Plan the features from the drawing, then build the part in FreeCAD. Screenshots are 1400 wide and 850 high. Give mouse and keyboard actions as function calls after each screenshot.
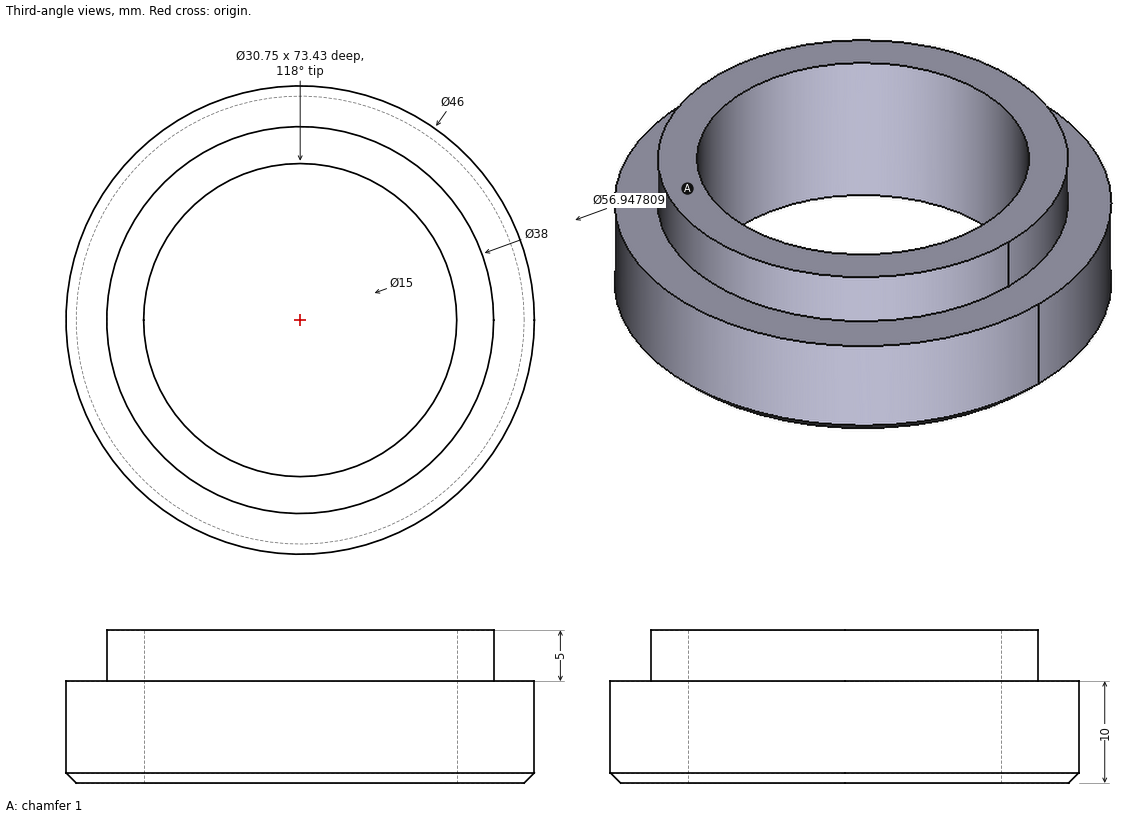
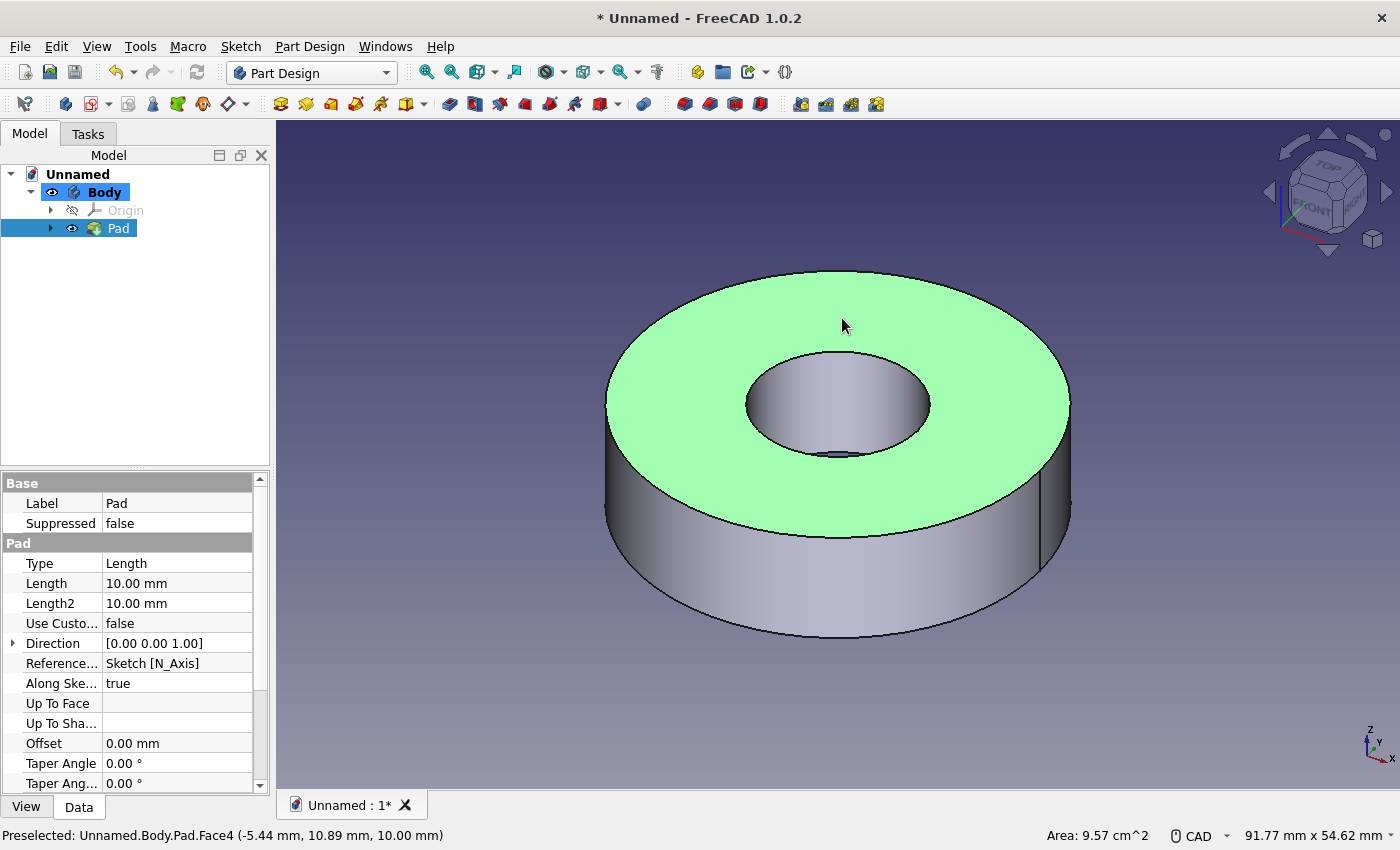
click(90, 104)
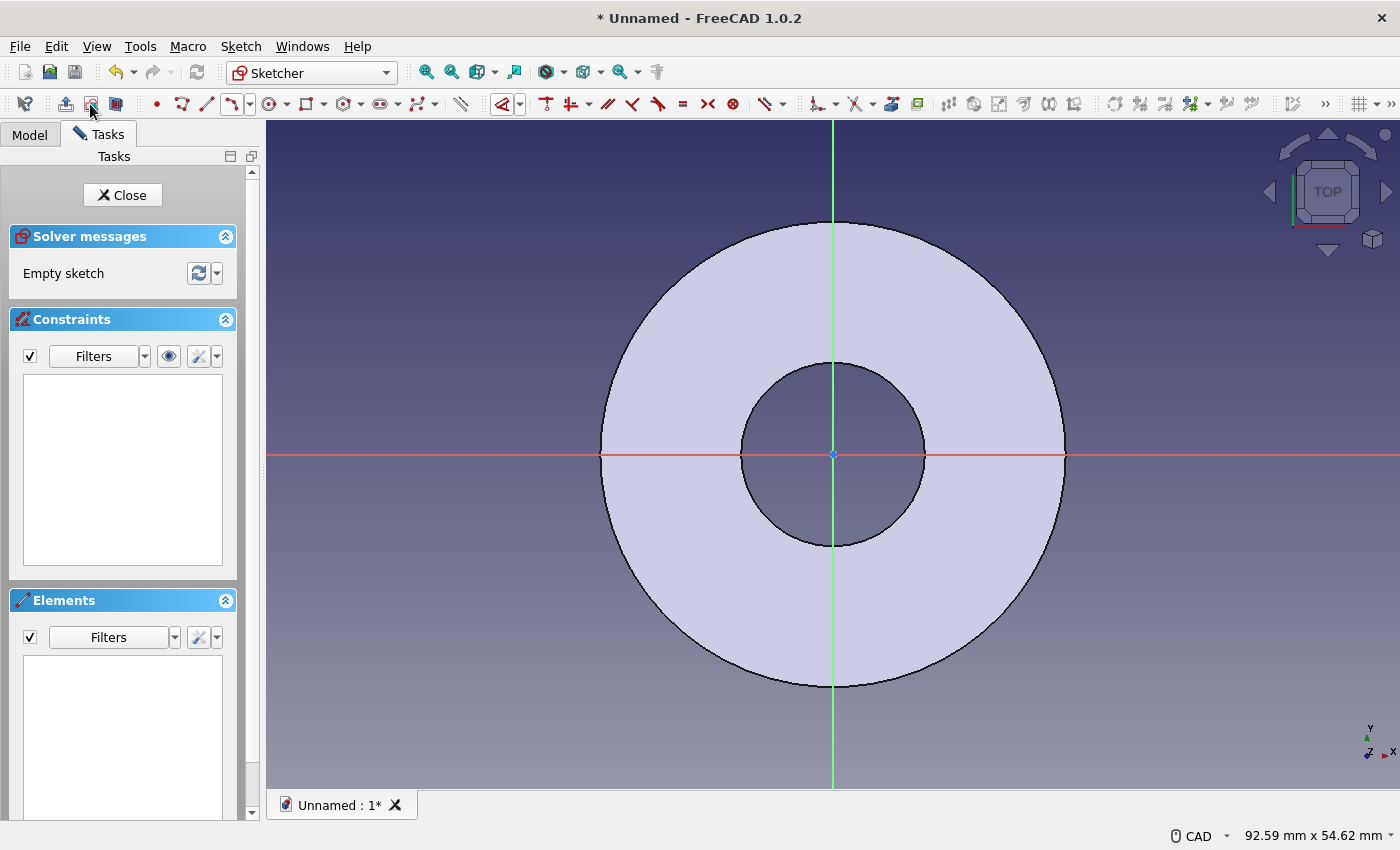
scroll(455, 455, down, 1)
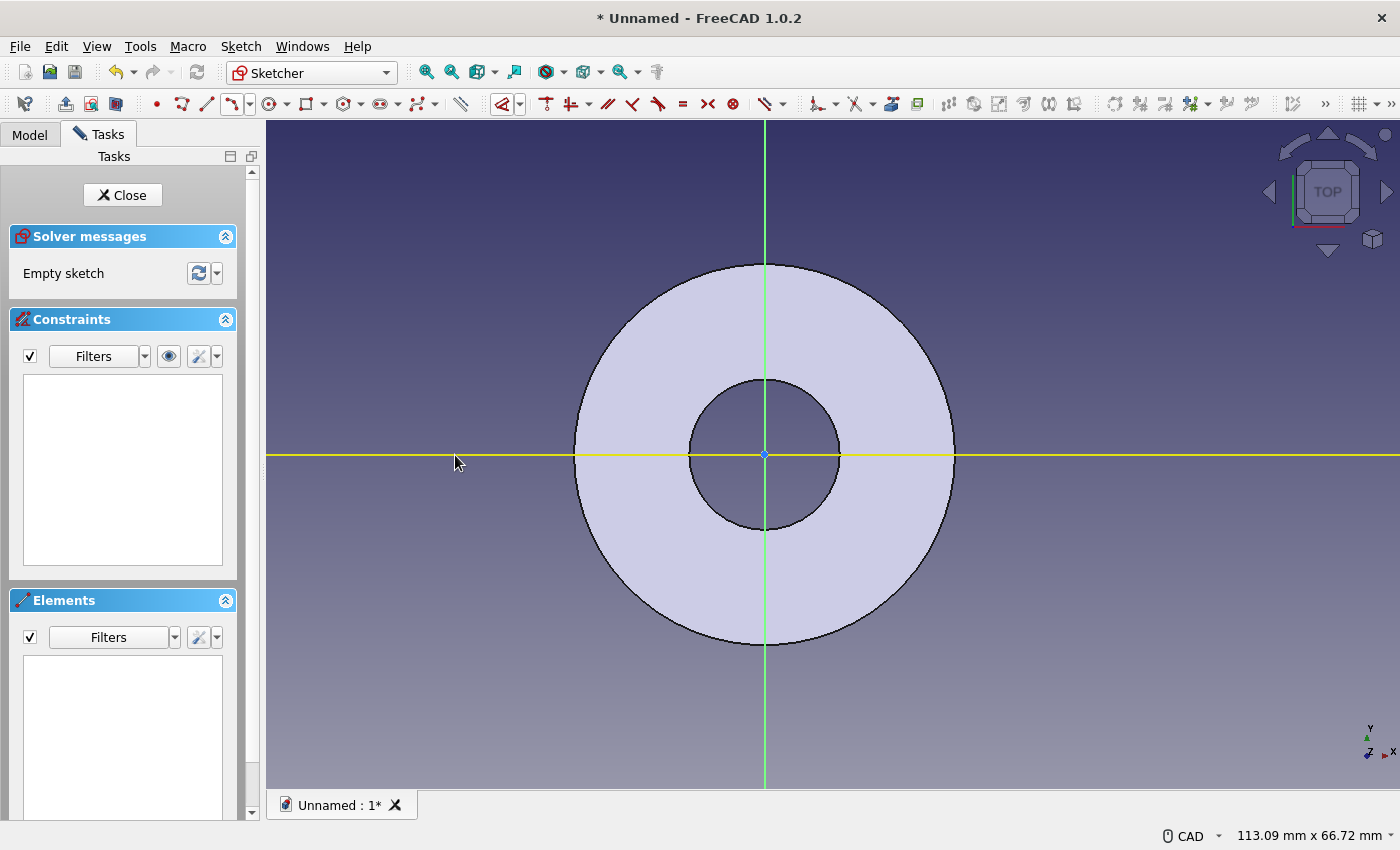
click(268, 104)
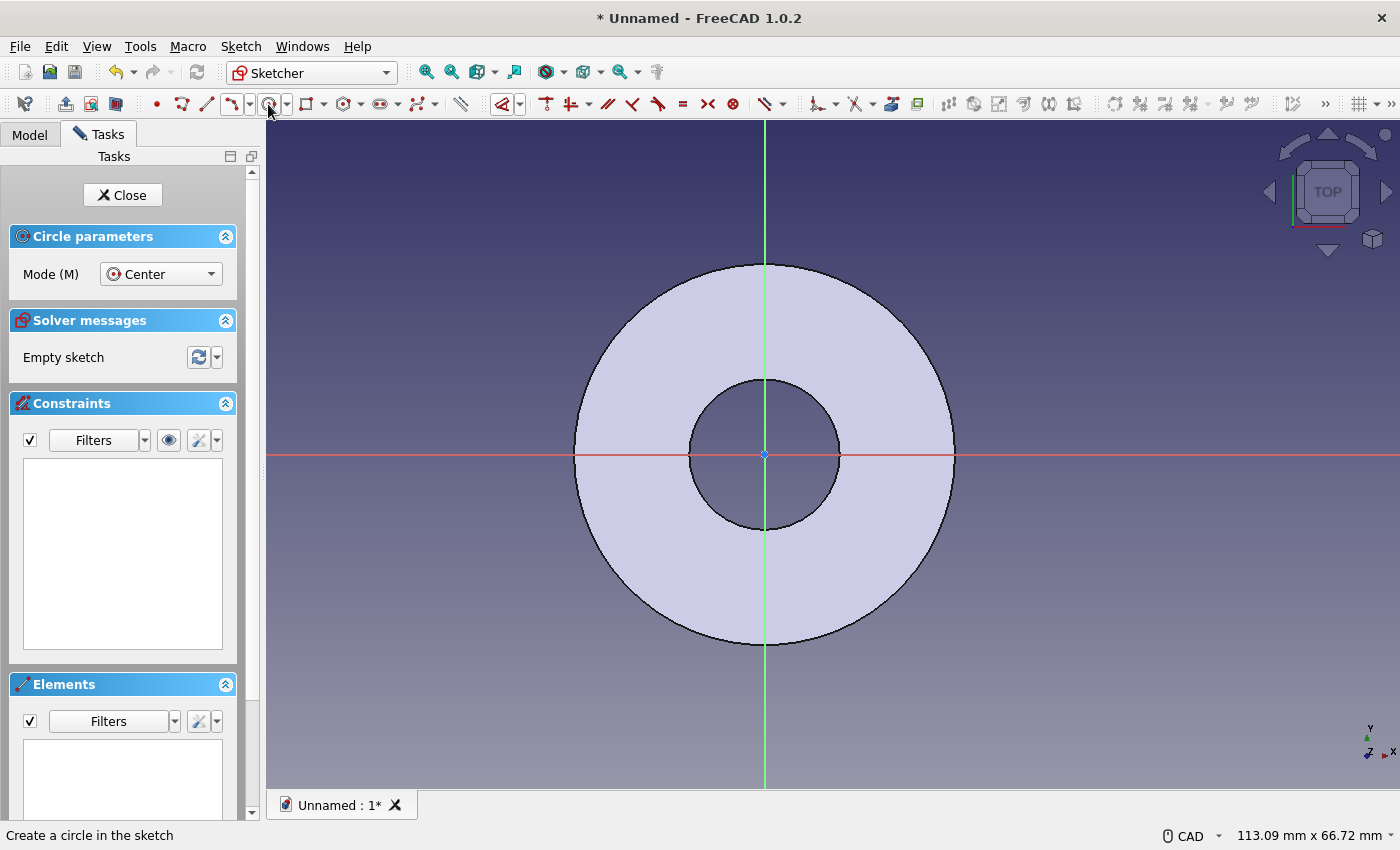
click(765, 455)
move(928, 292)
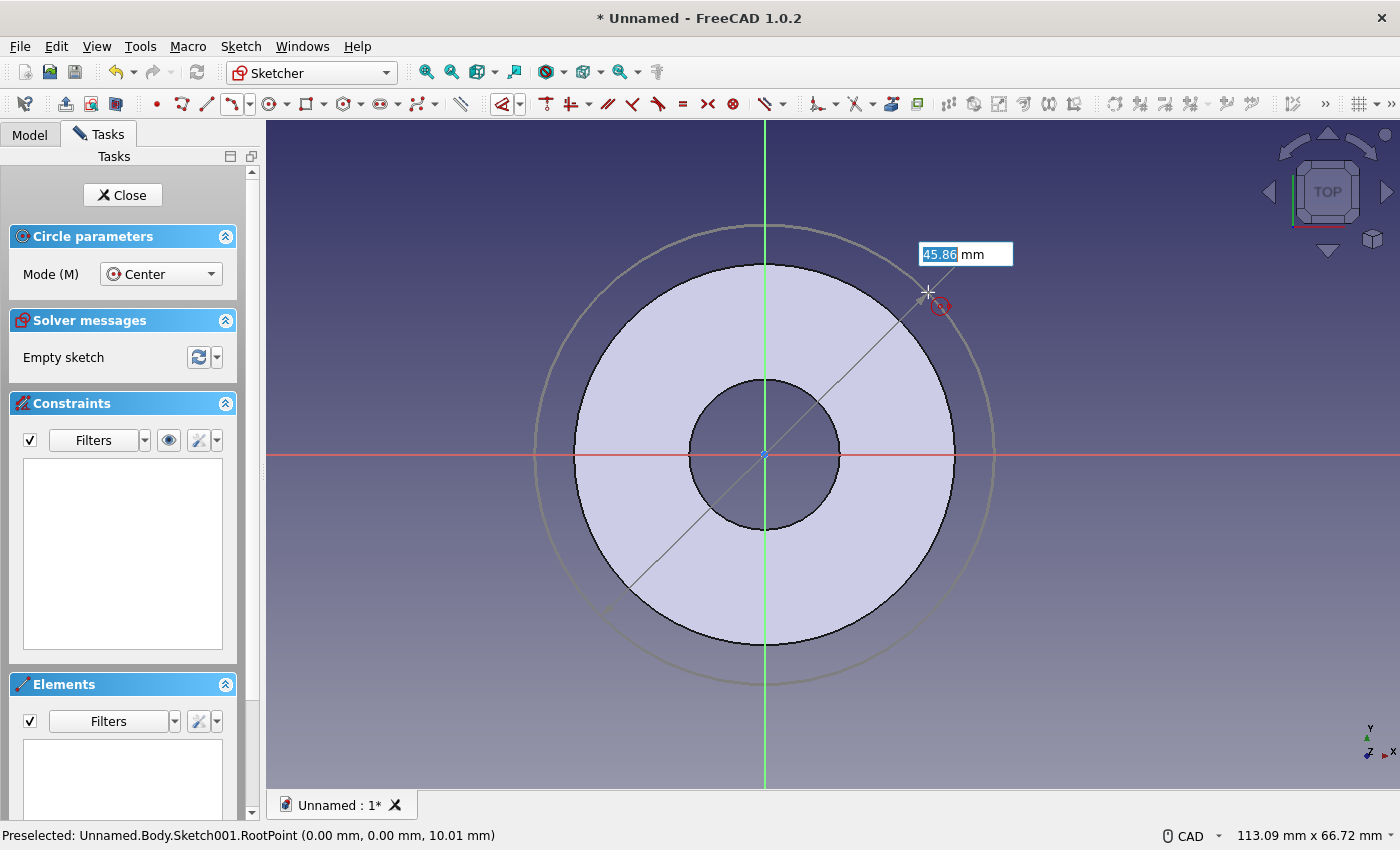
text(46)
key(Return)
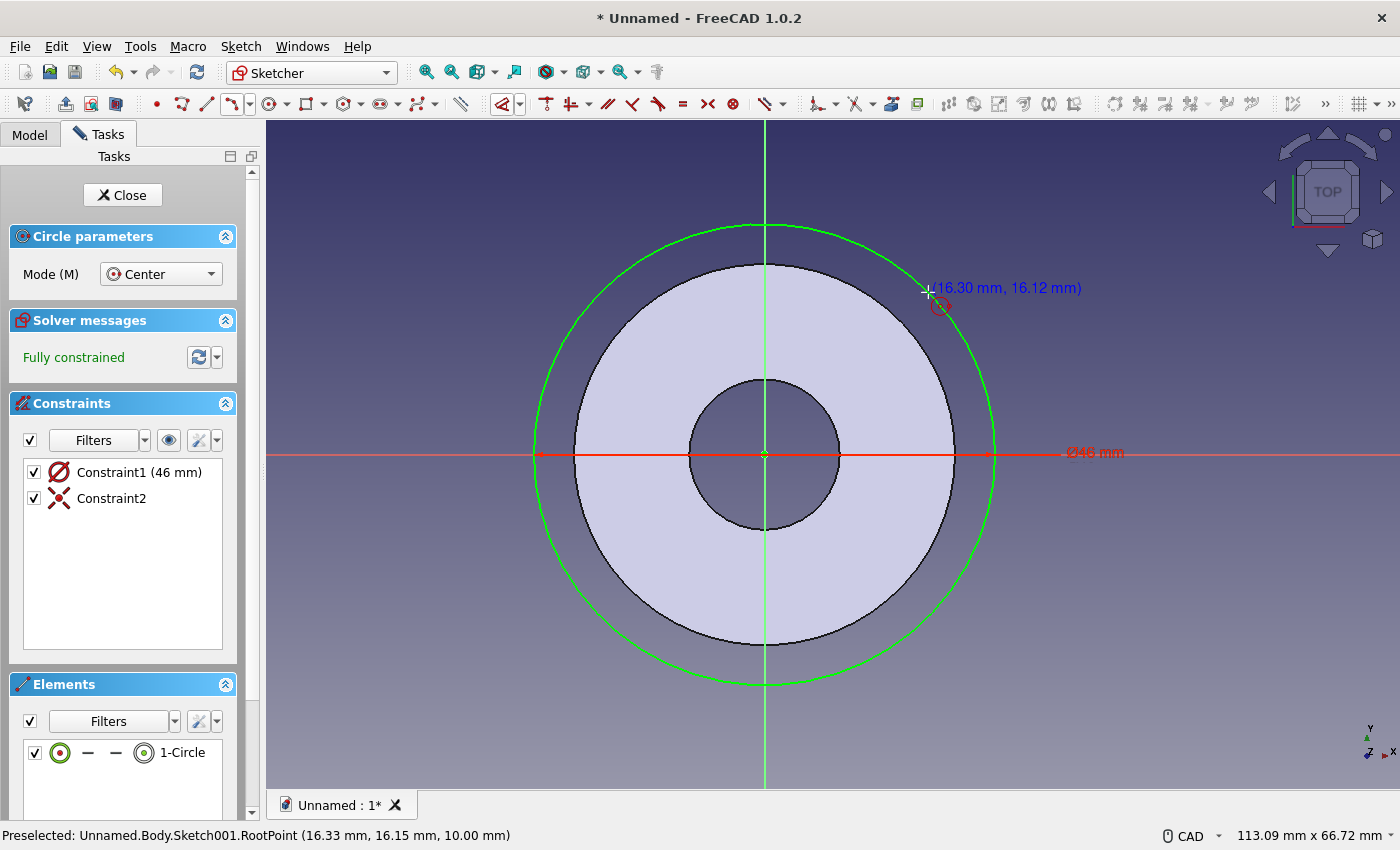
click(765, 455)
move(818, 402)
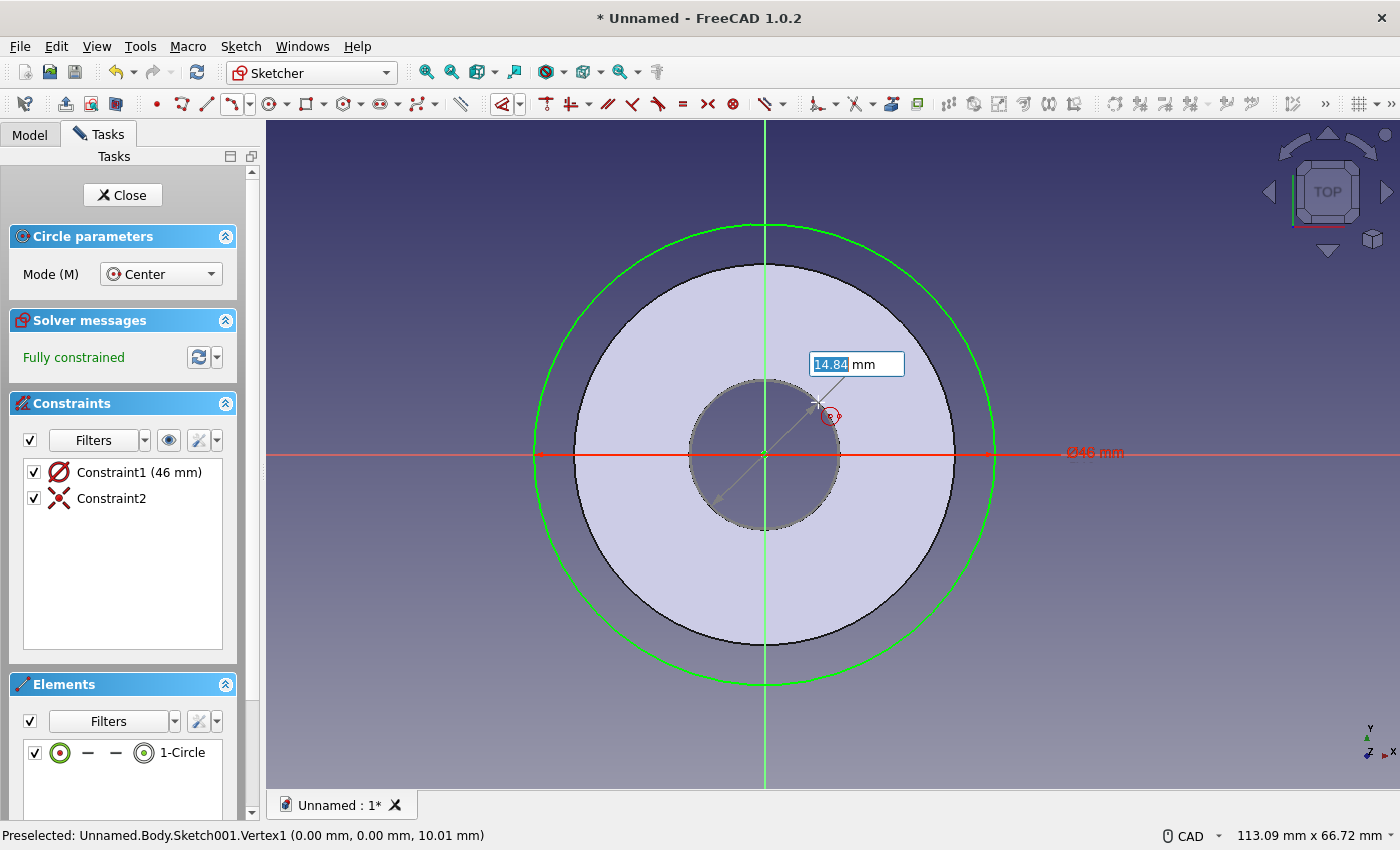
text(15)
key(Return)
key(Escape)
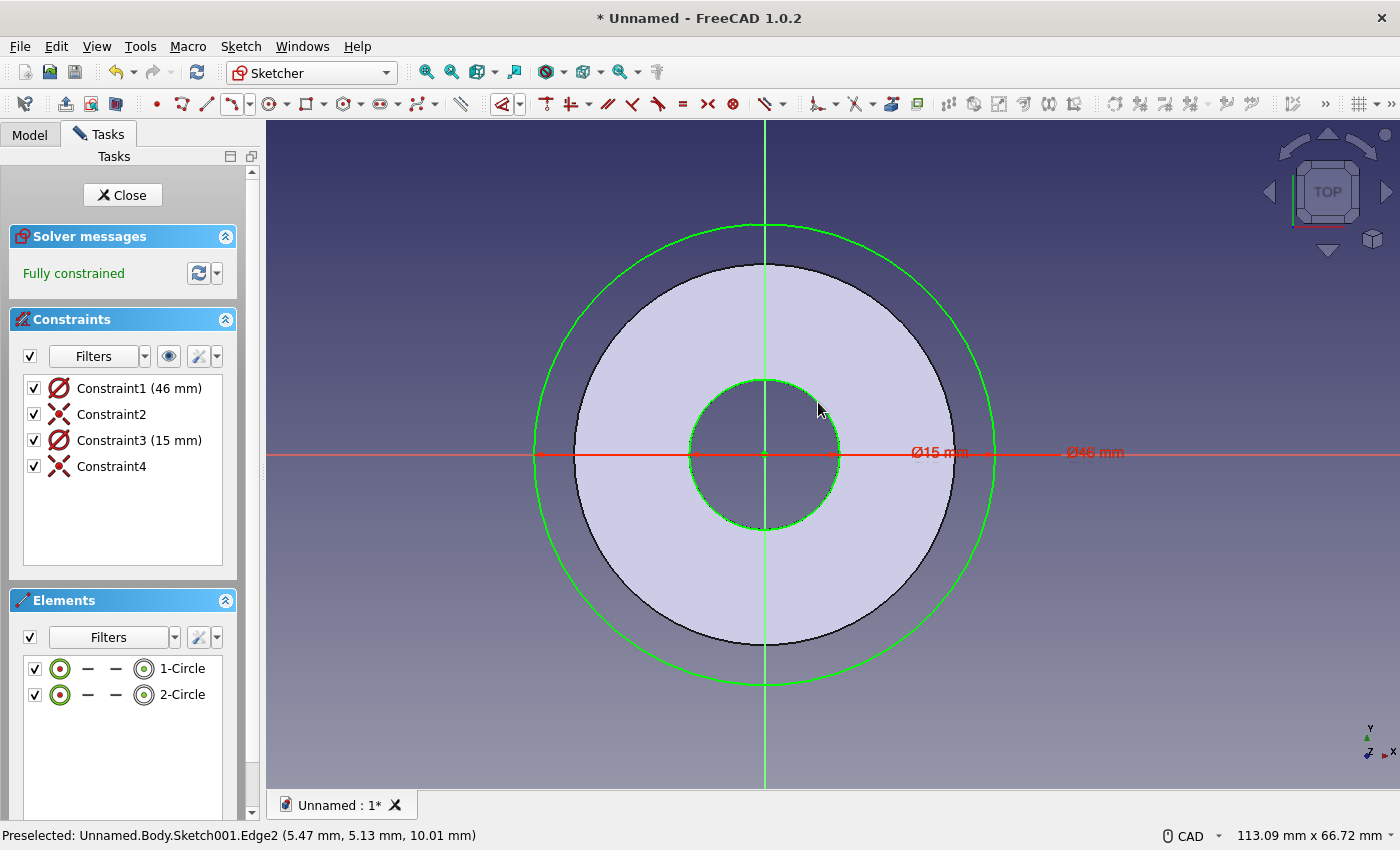
click(123, 195)